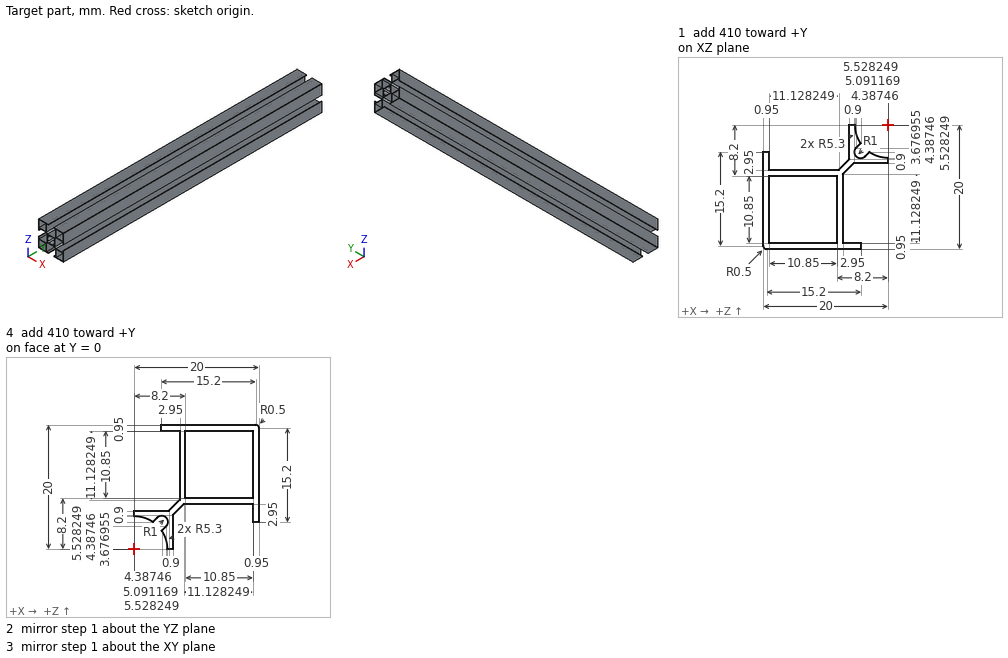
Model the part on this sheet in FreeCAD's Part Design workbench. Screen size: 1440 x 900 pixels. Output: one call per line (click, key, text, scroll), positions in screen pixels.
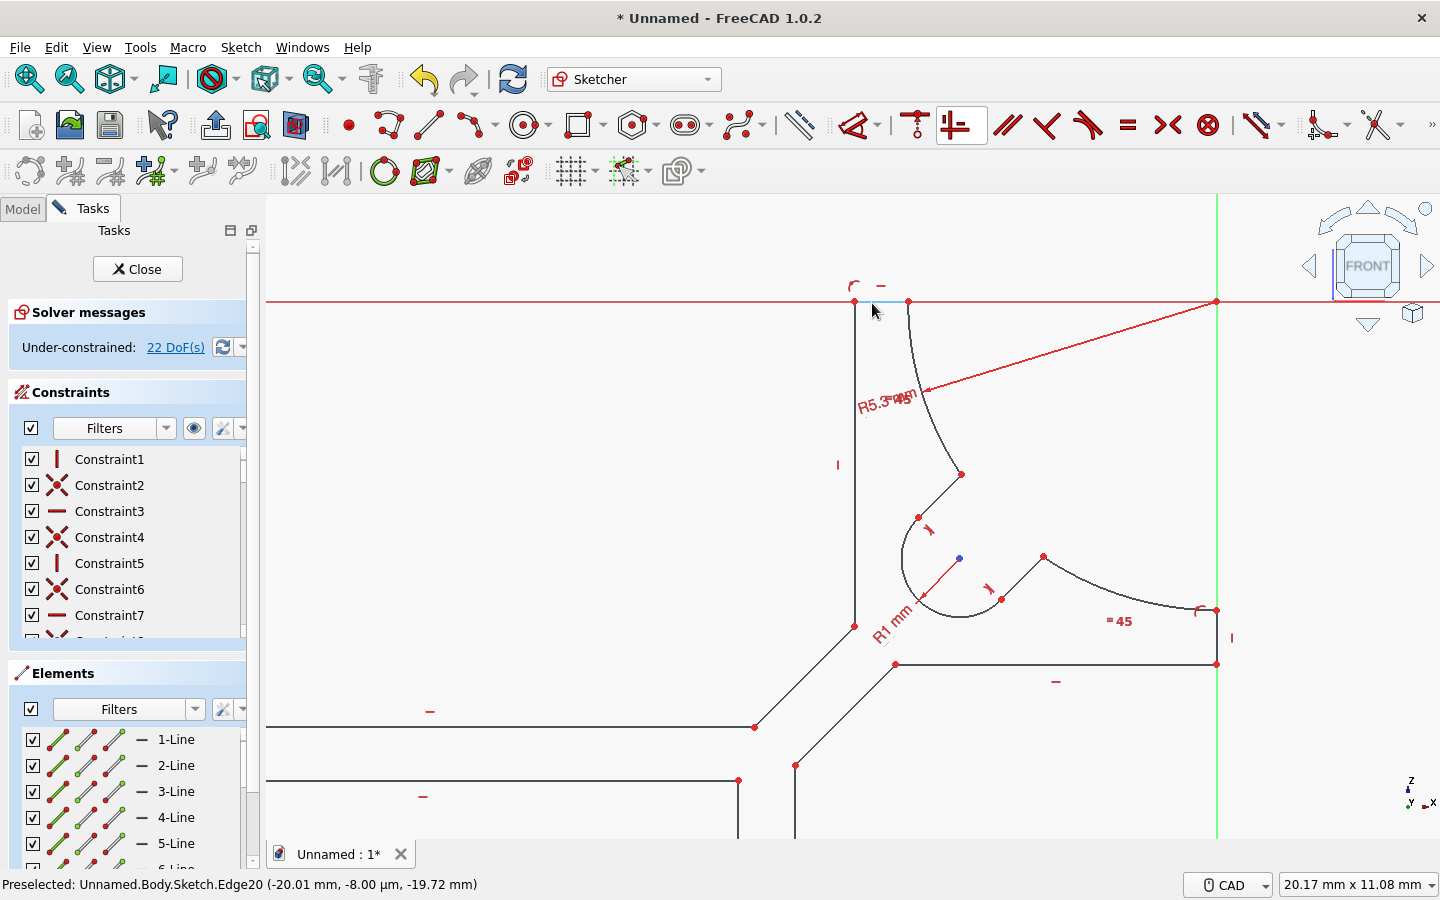
click(871, 302)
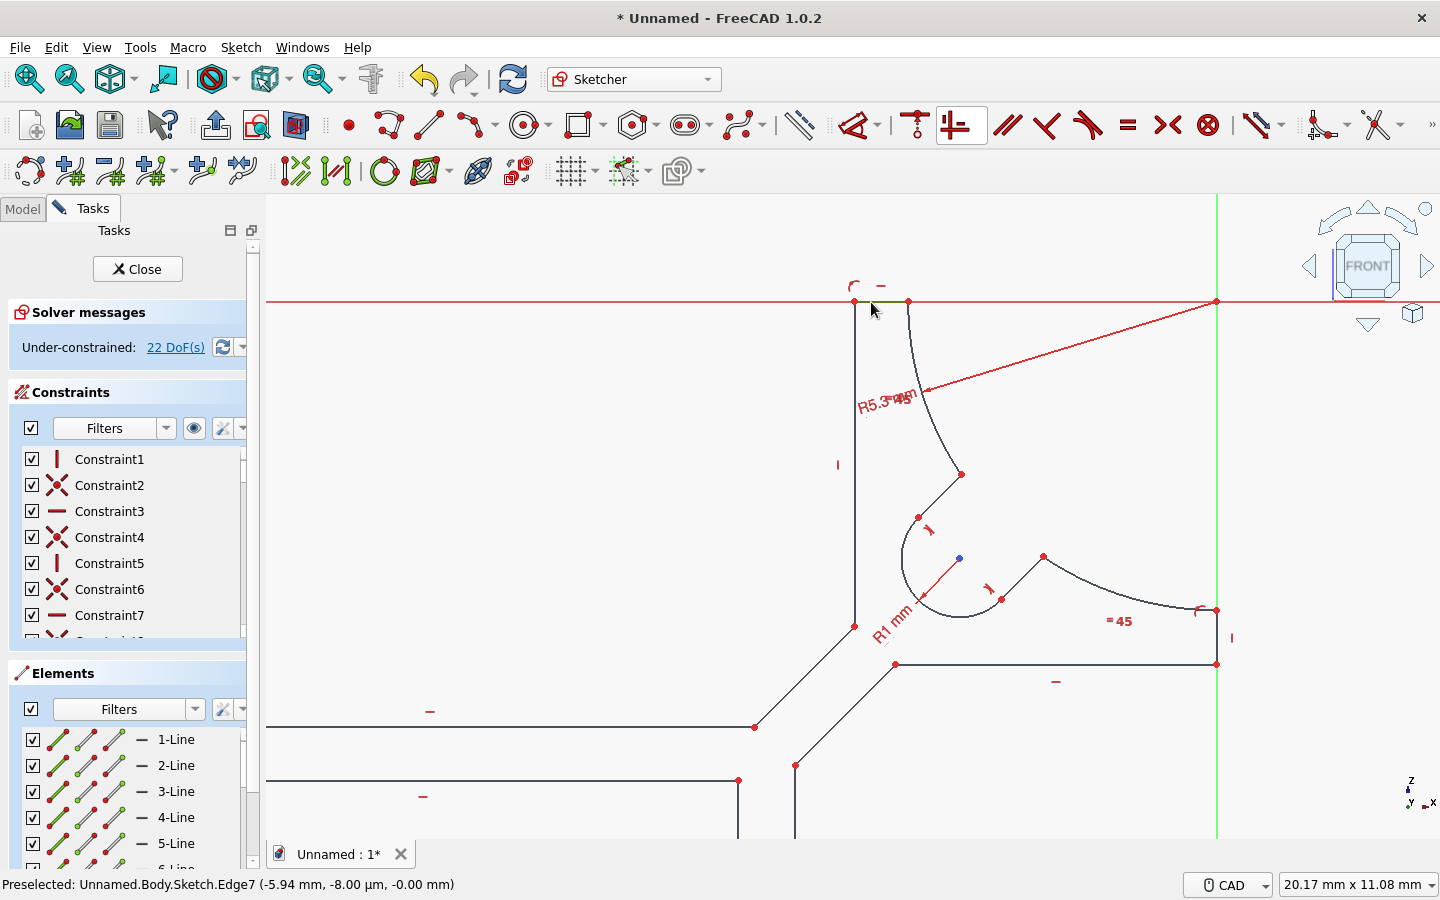
click(880, 126)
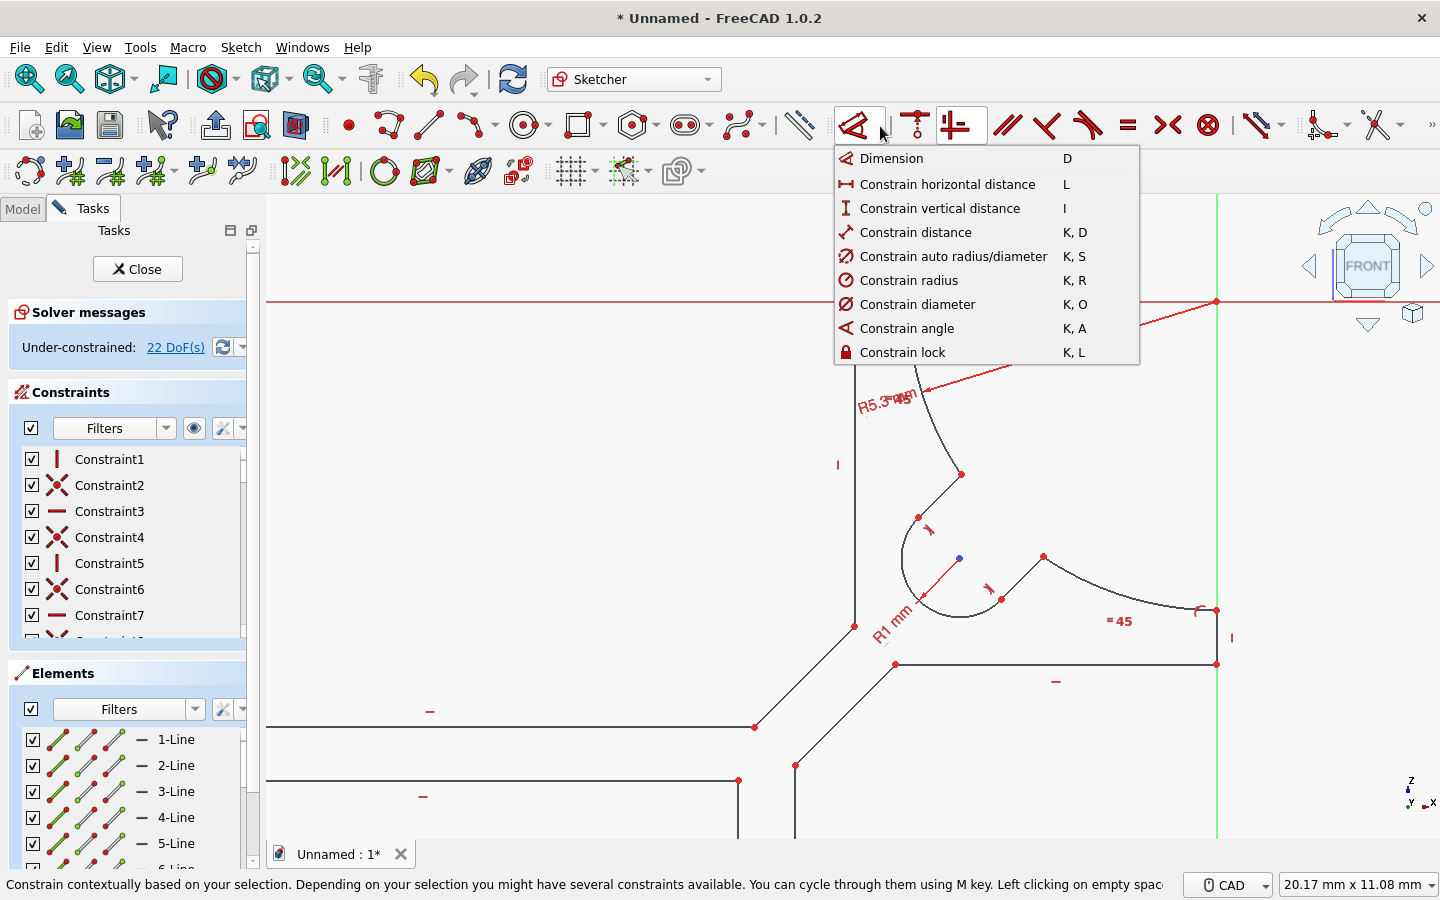
click(987, 184)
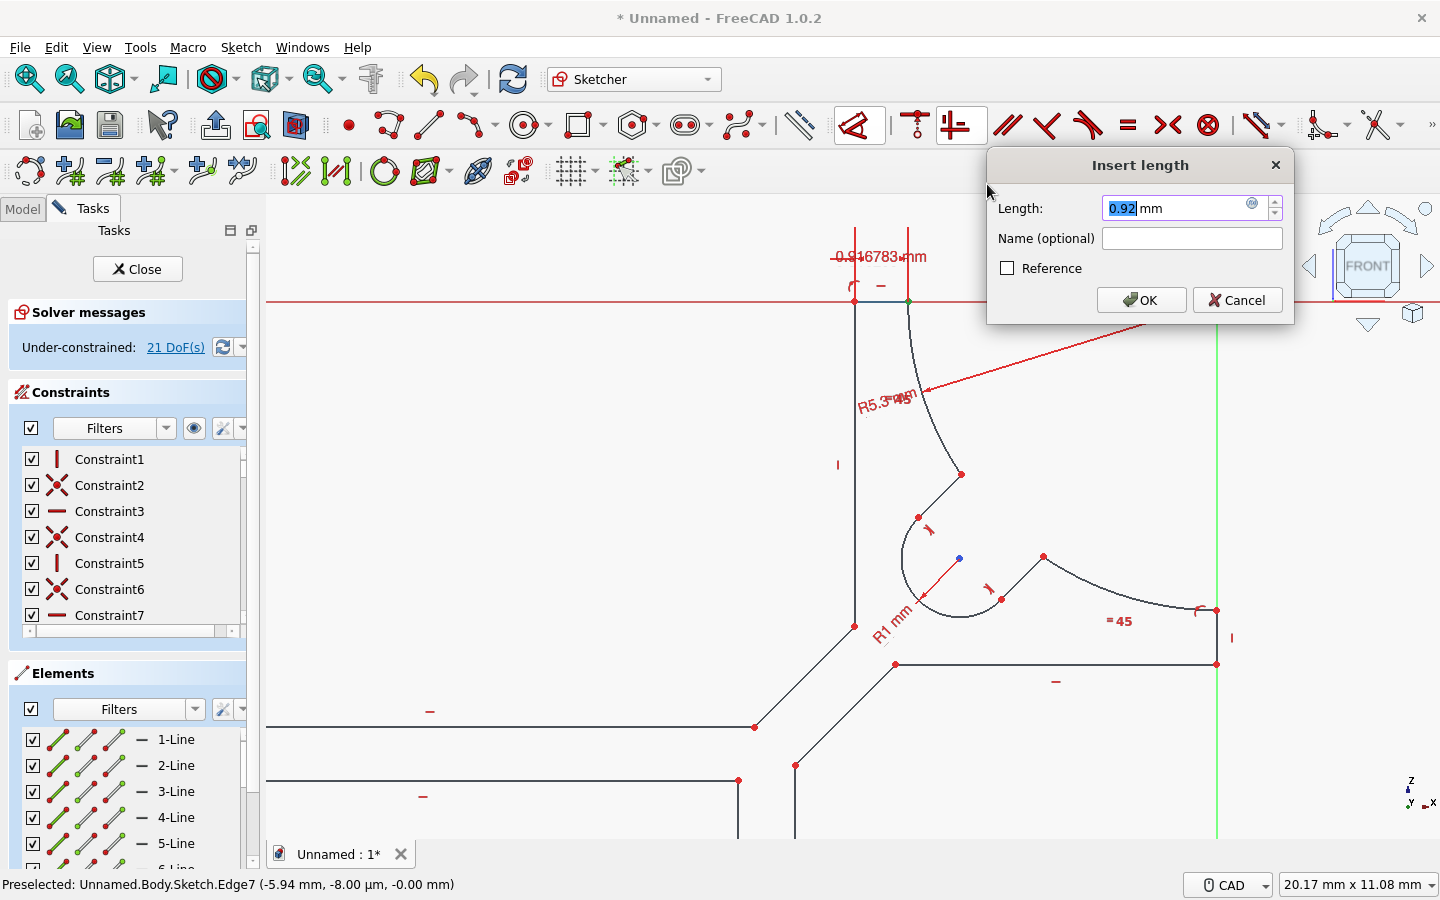
text(0.9)
key(Return)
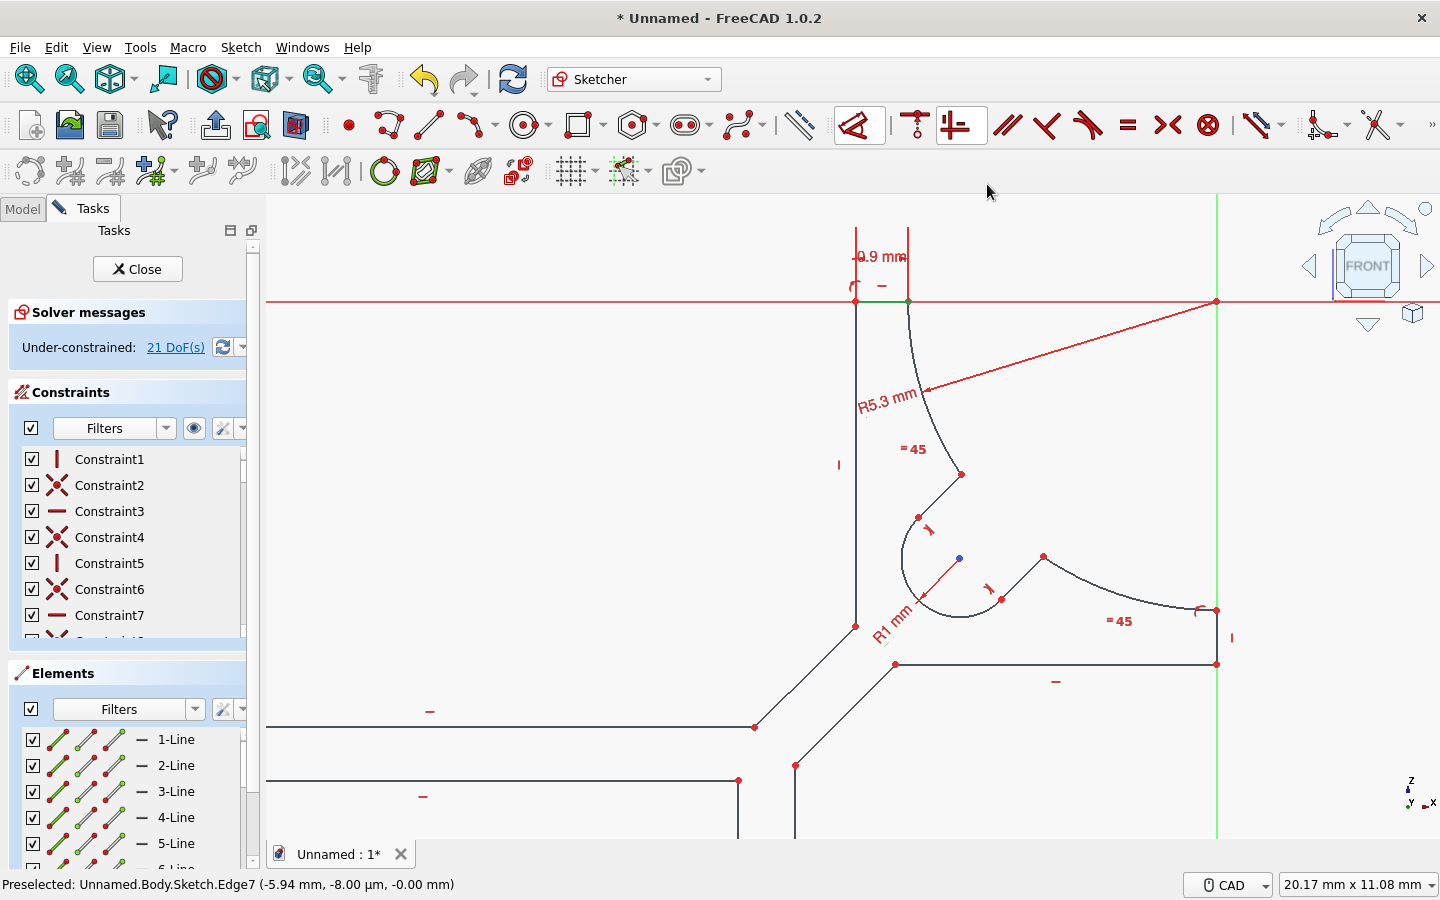
click(1217, 627)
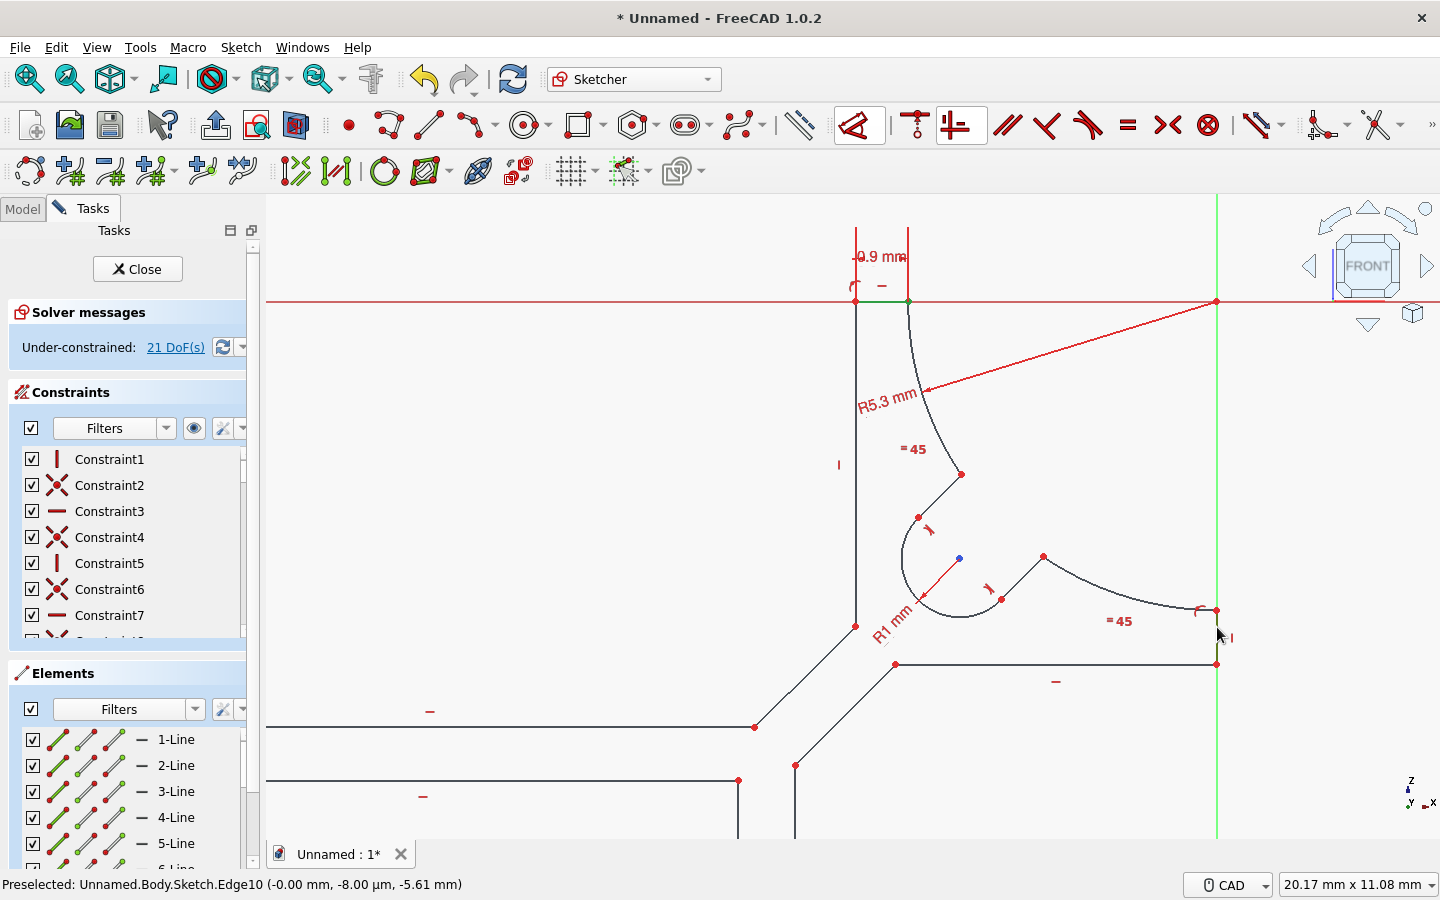
key(i)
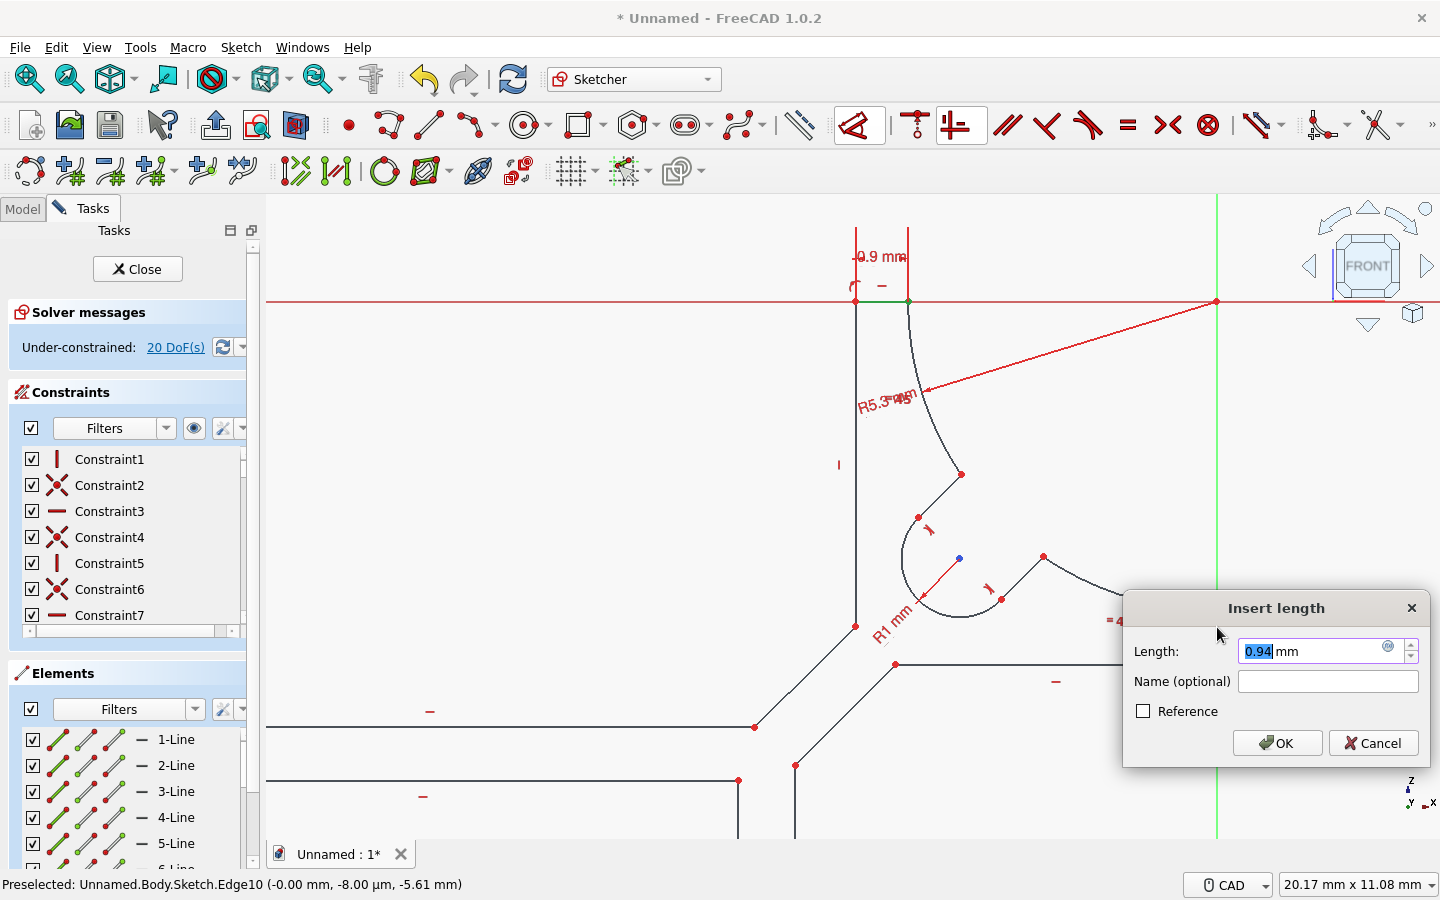
text(0.9)
key(Return)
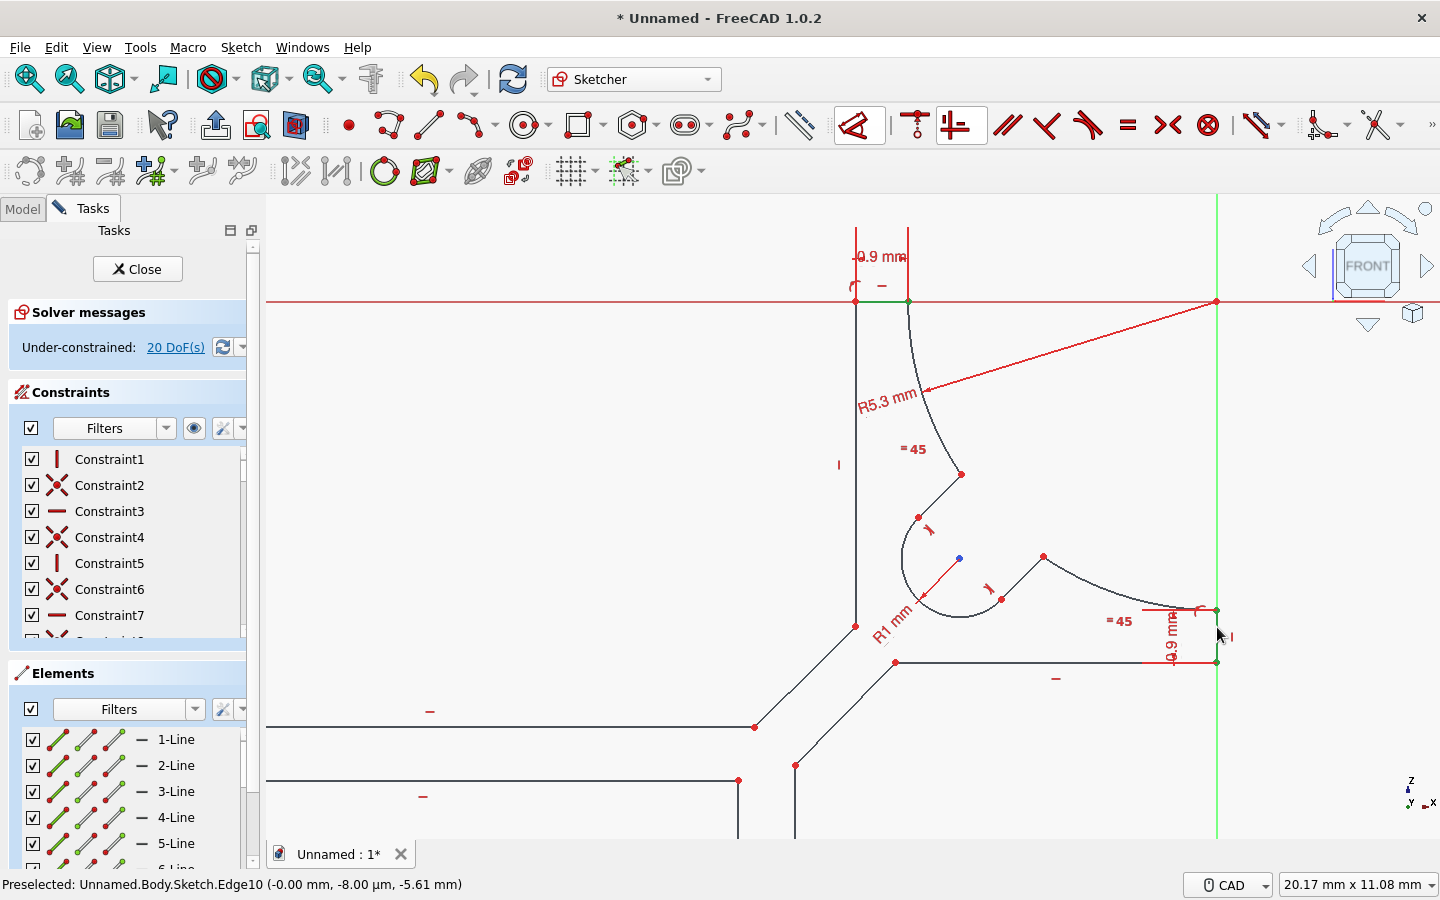
scroll(872, 303, down, 5)